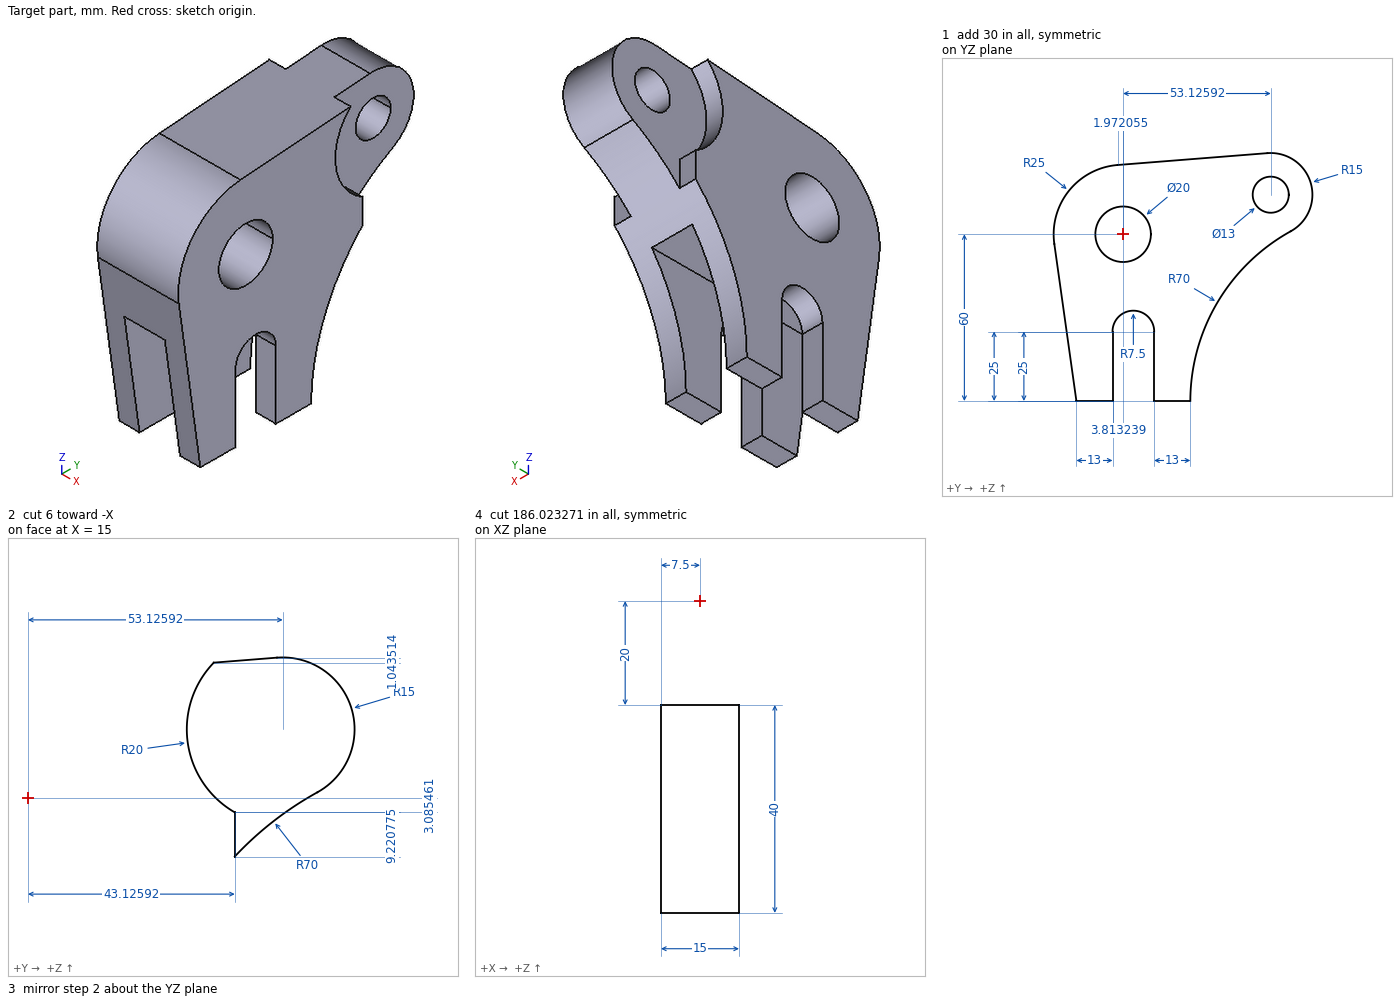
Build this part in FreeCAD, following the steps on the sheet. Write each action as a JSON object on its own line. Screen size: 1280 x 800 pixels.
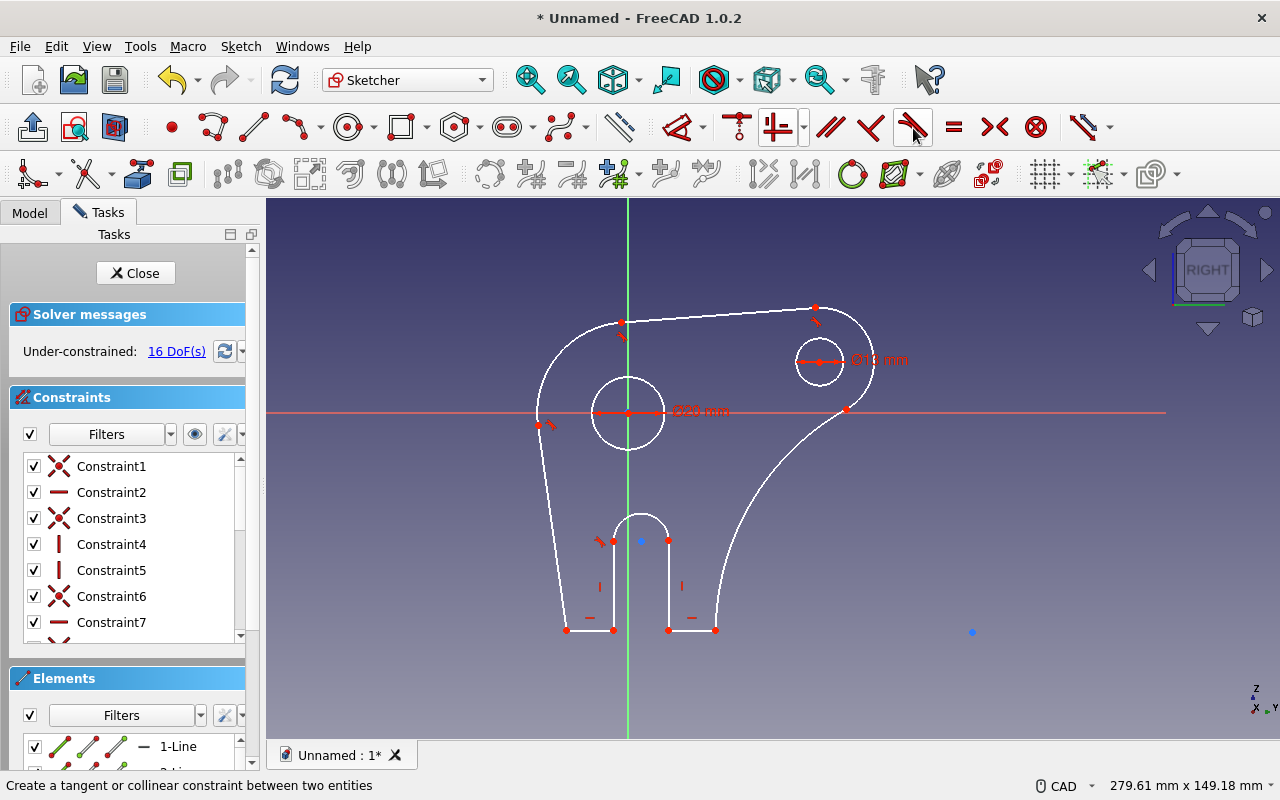
{"action": "left_click", "coordinate": [669, 568]}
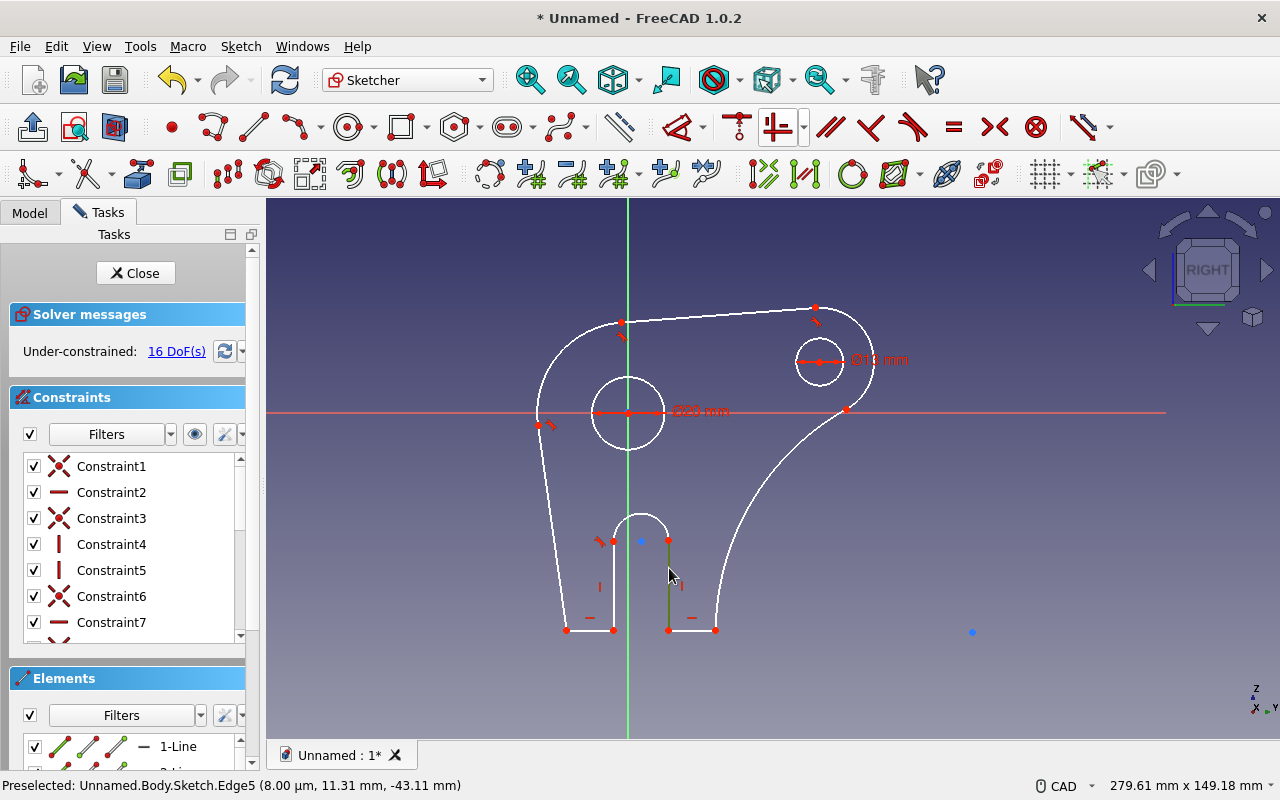
{"action": "left_click", "coordinate": [657, 519]}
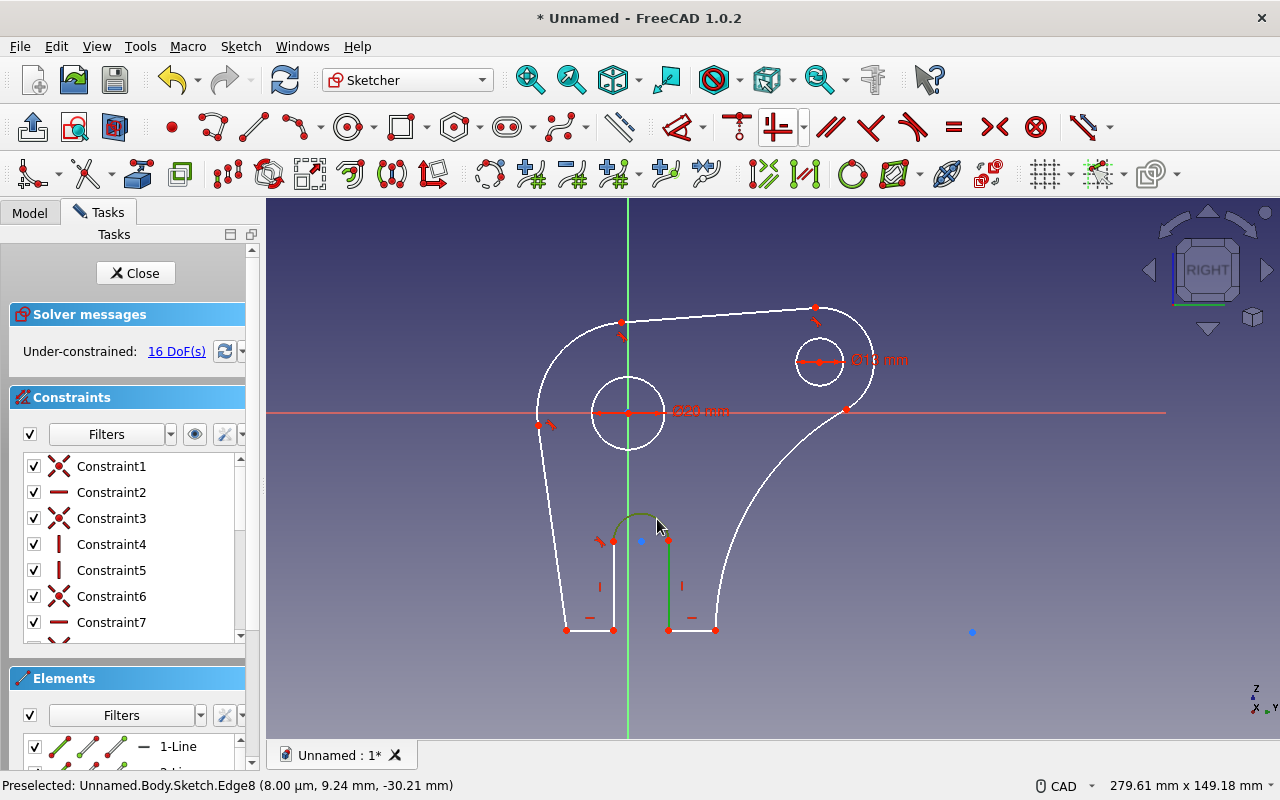
{"action": "left_click", "coordinate": [913, 128]}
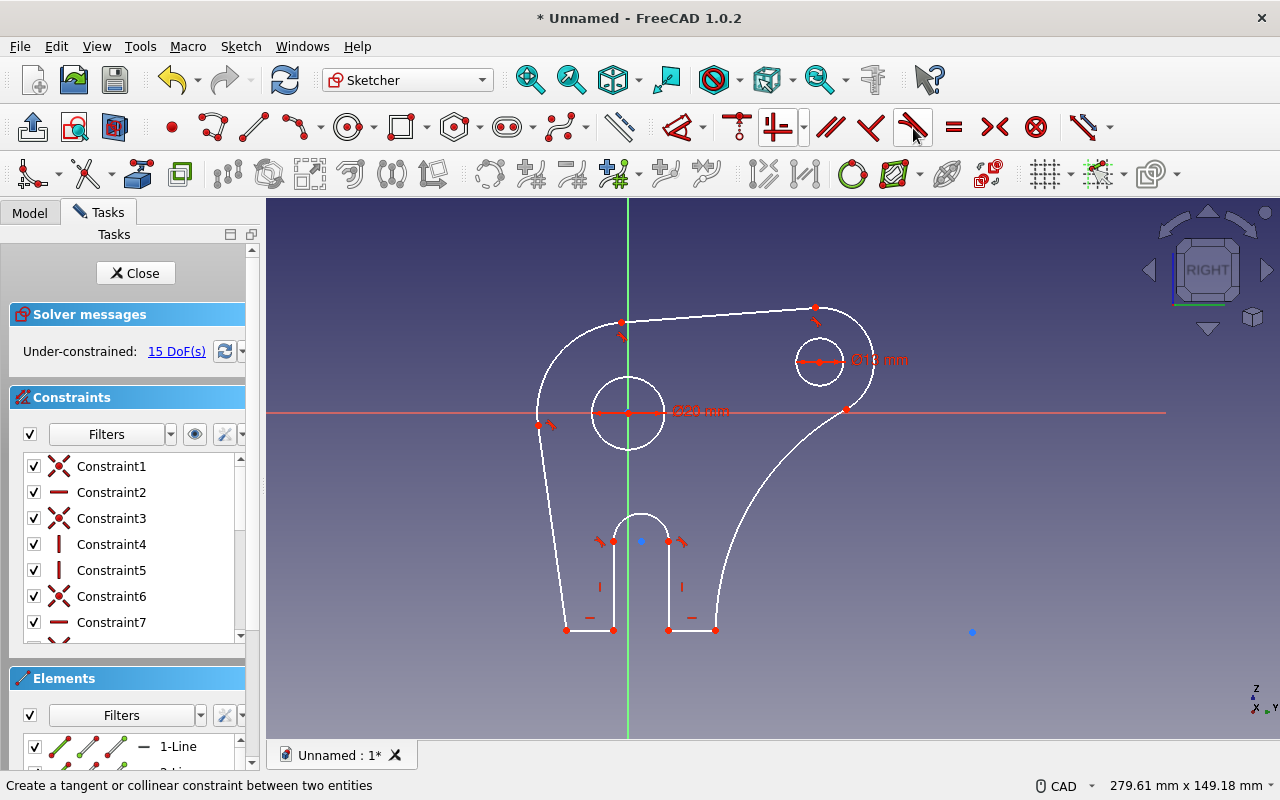
{"action": "left_click", "coordinate": [783, 459]}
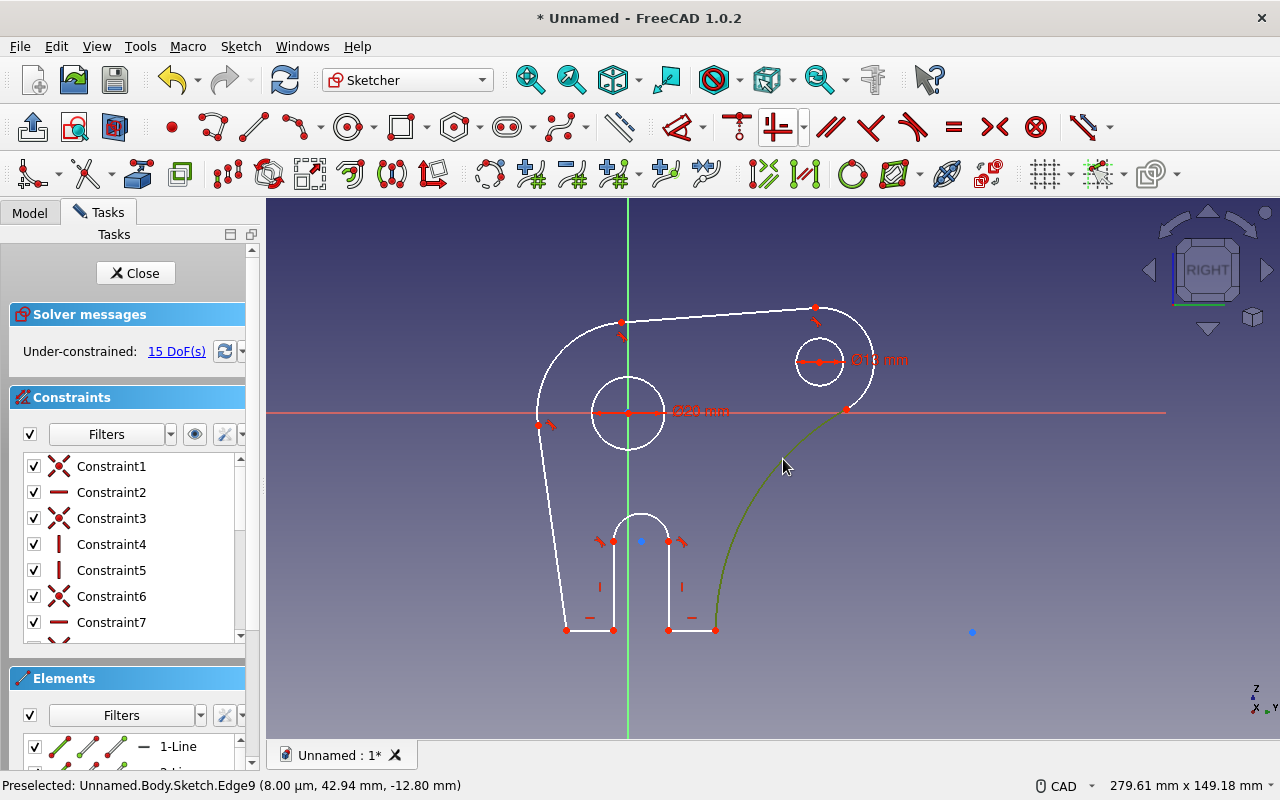
{"action": "left_click", "coordinate": [872, 375]}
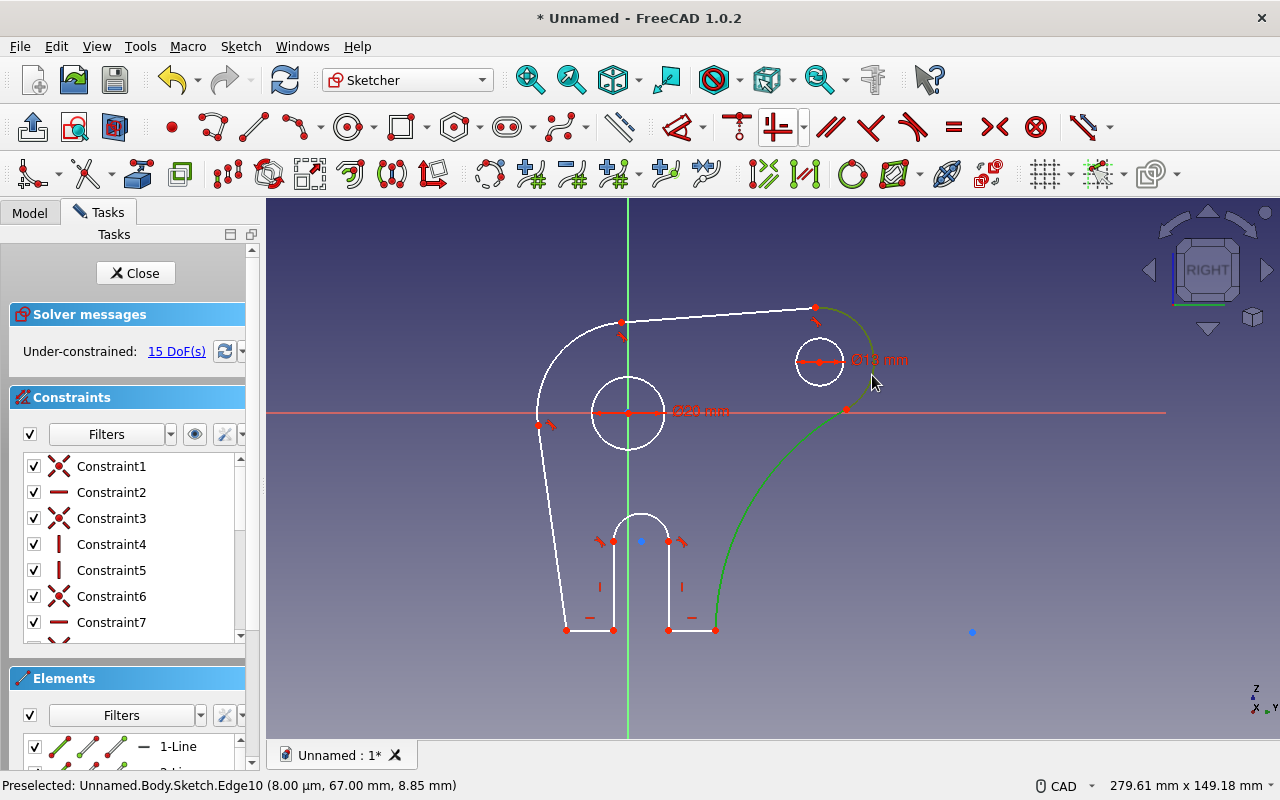
{"action": "left_click", "coordinate": [913, 128]}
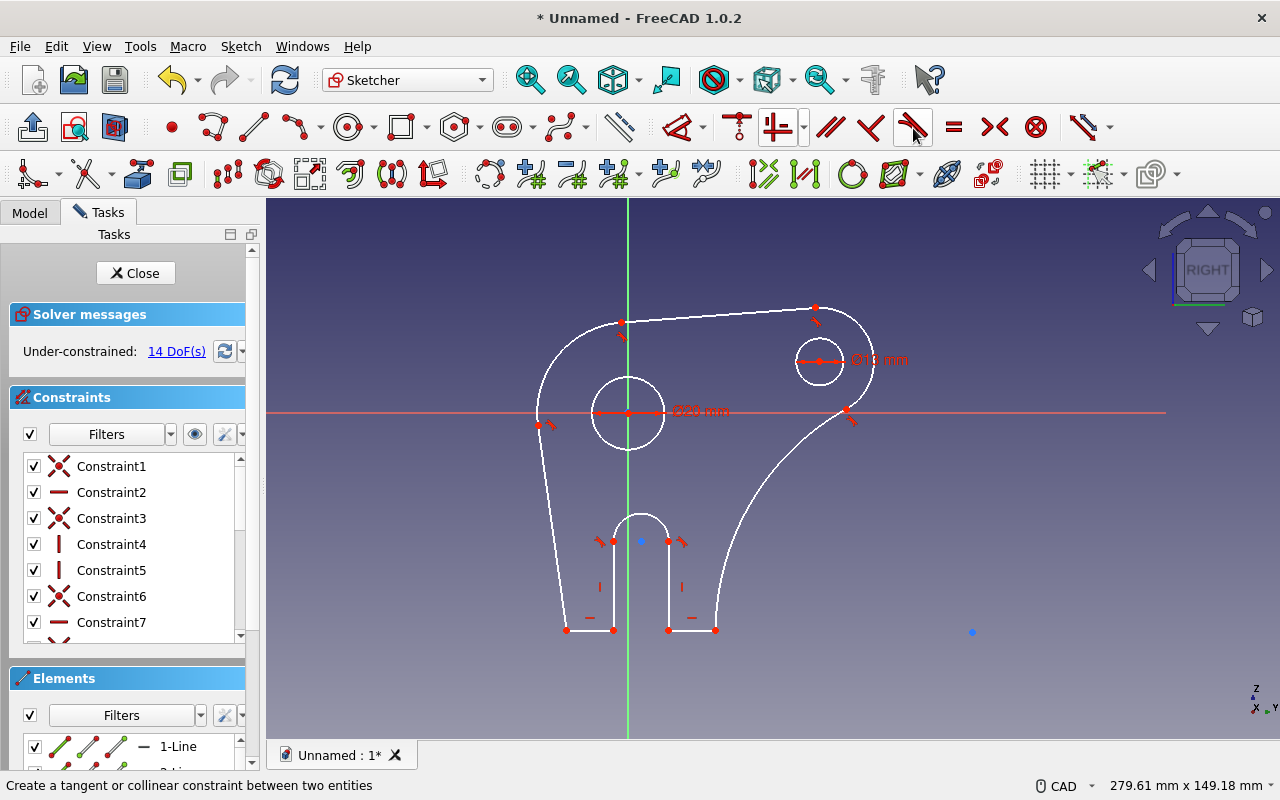
{"action": "scroll", "coordinate": [628, 413], "scroll_direction": "up", "scroll_amount": 3}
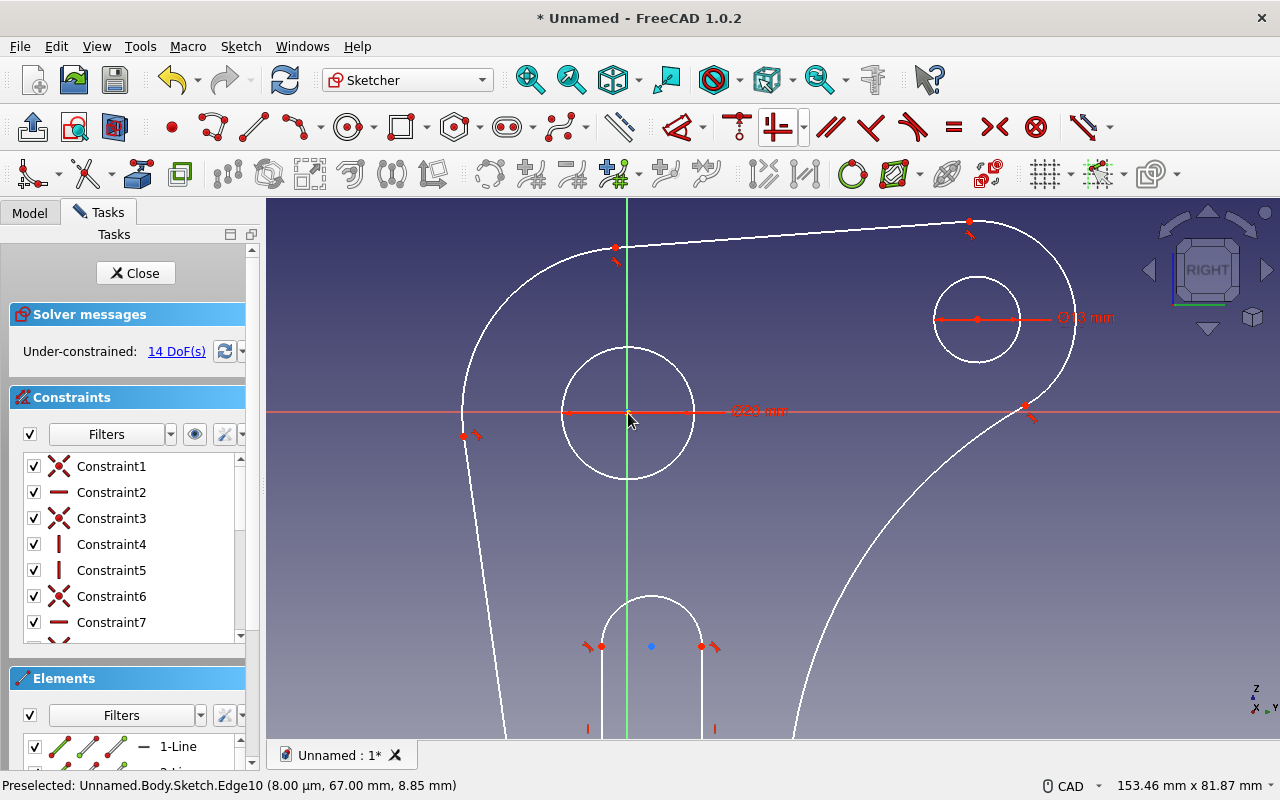
{"action": "left_click_drag", "start_coordinate": [617, 402], "coordinate": [638, 423]}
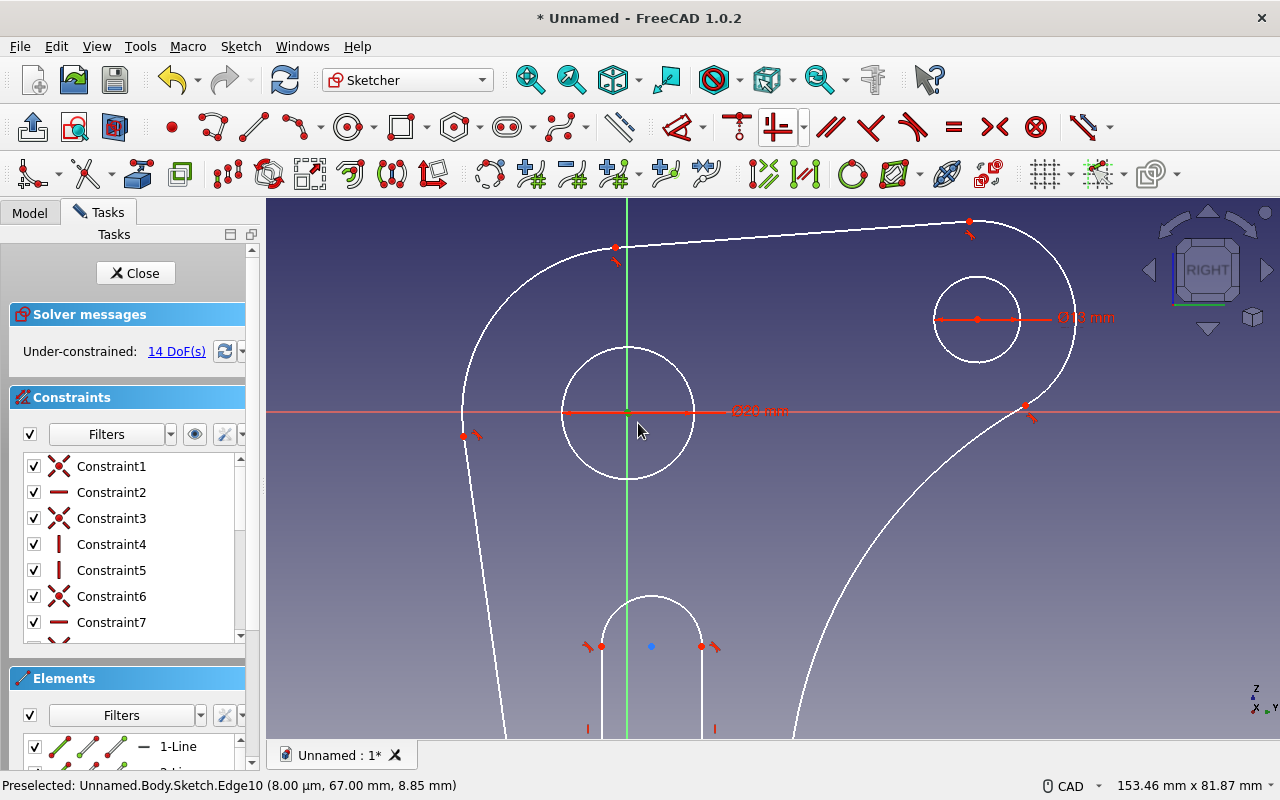
{"action": "left_click", "coordinate": [737, 128]}